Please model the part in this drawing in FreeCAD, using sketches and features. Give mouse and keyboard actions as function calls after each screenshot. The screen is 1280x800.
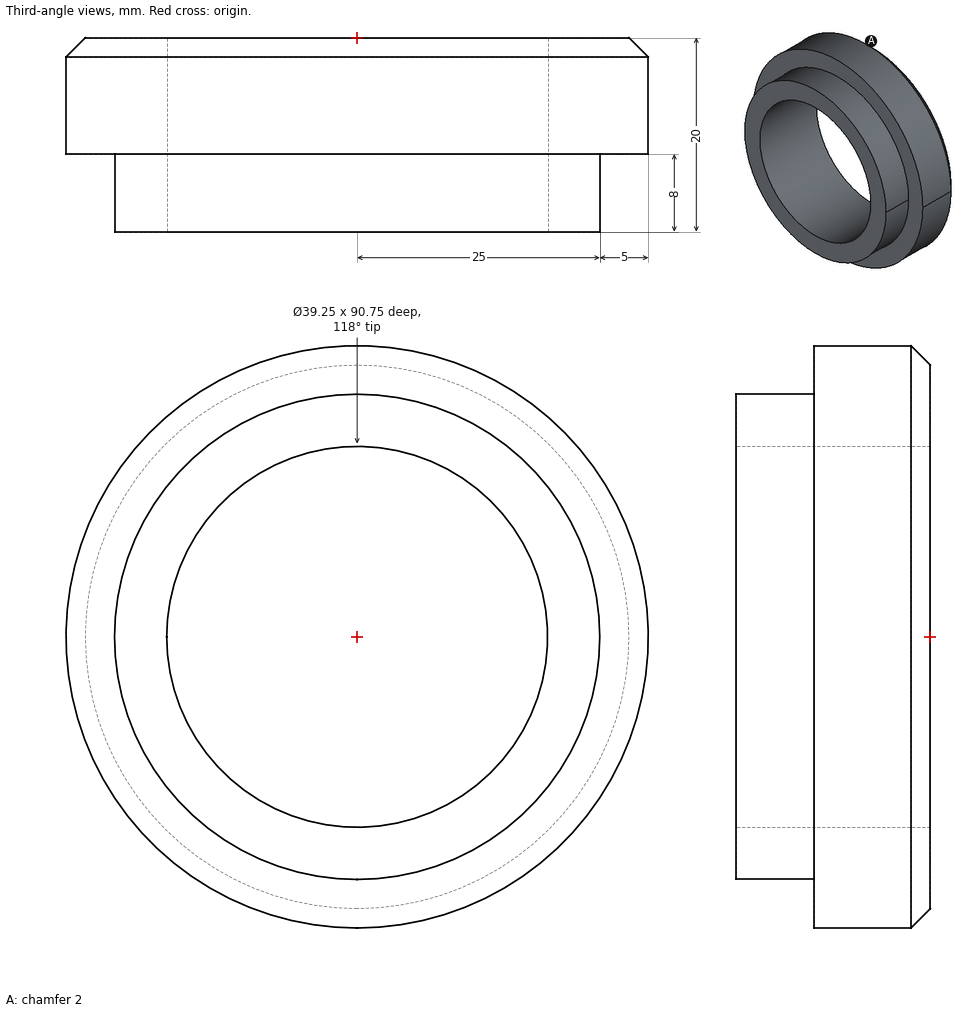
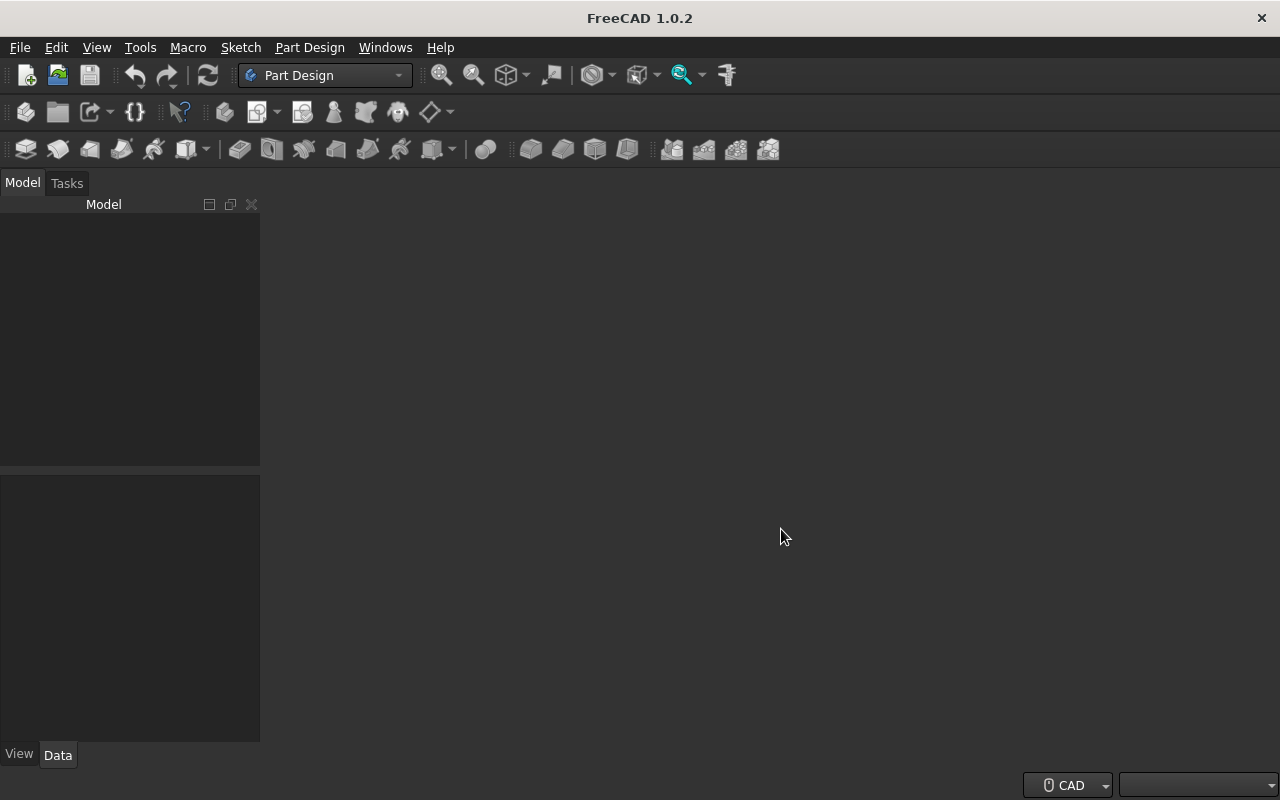
click(26, 76)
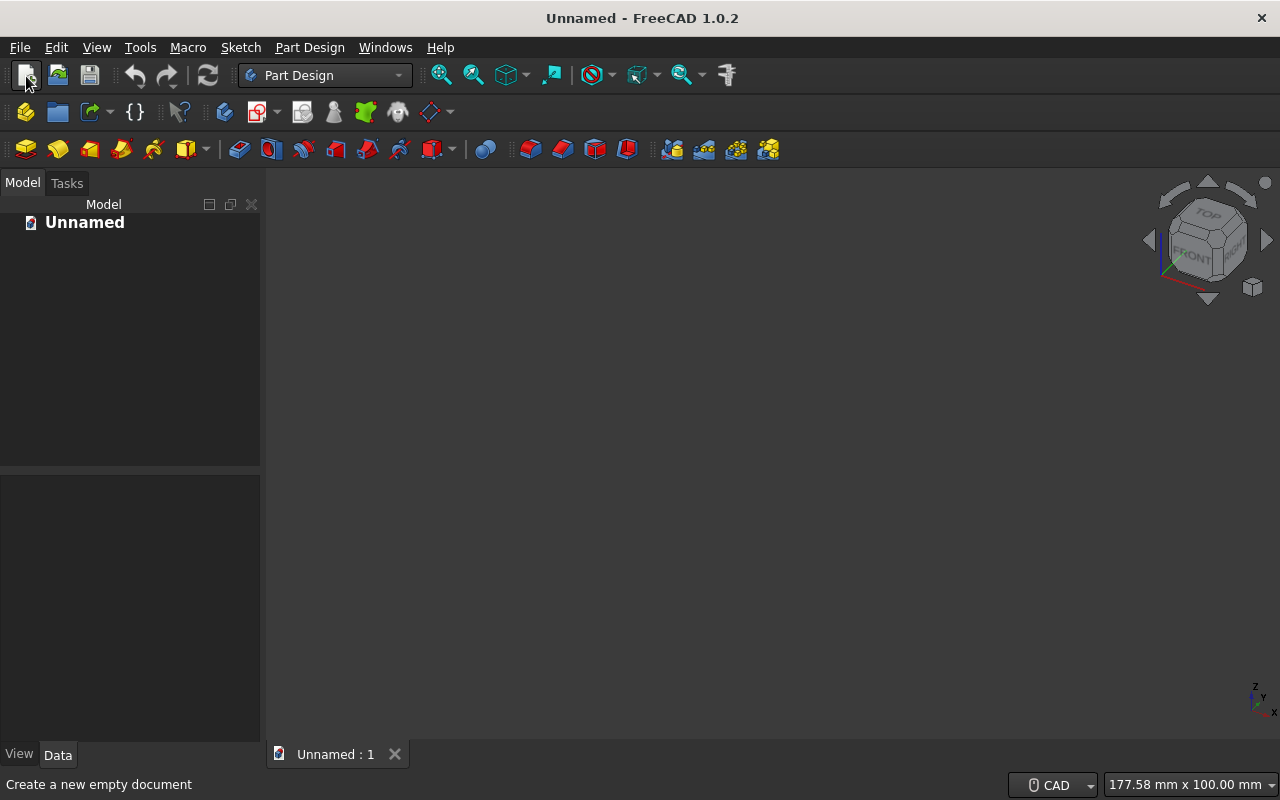
click(258, 112)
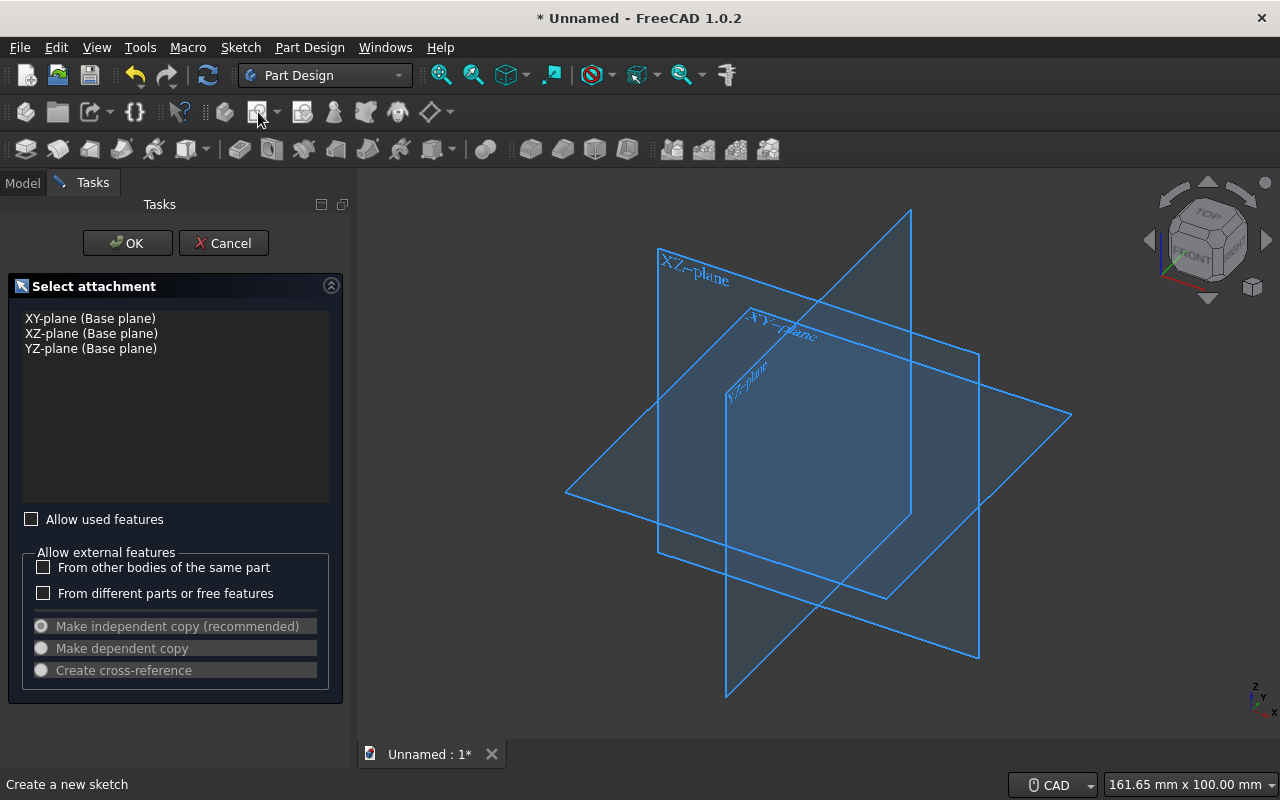
click(82, 318)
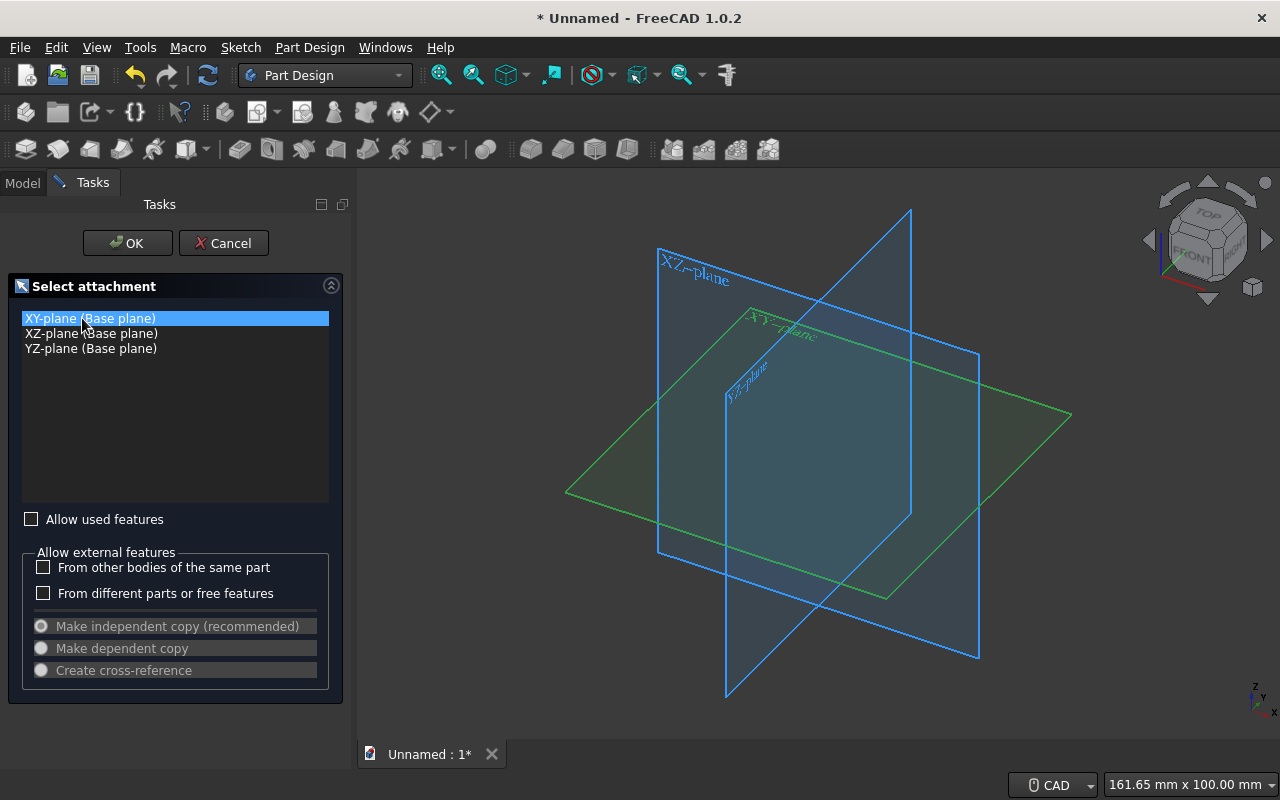
click(128, 243)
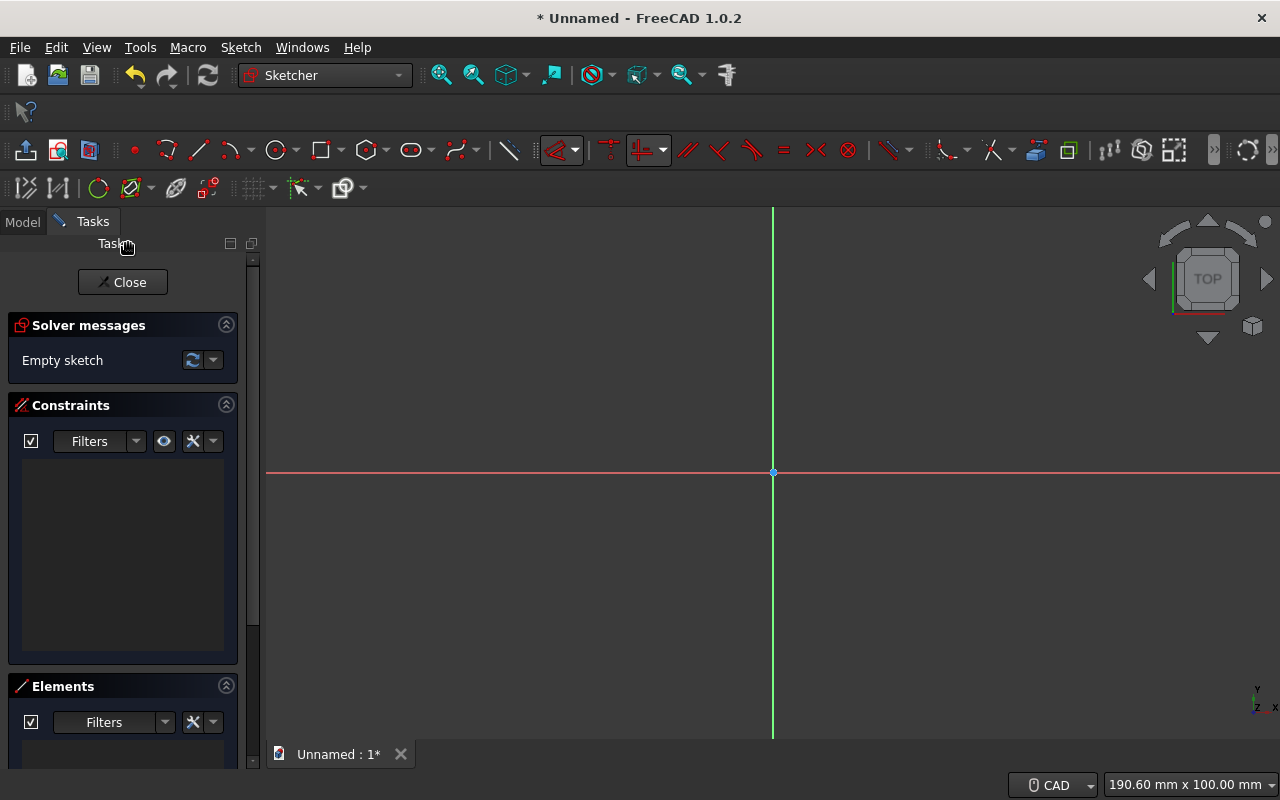
scroll(917, 549, up, 6)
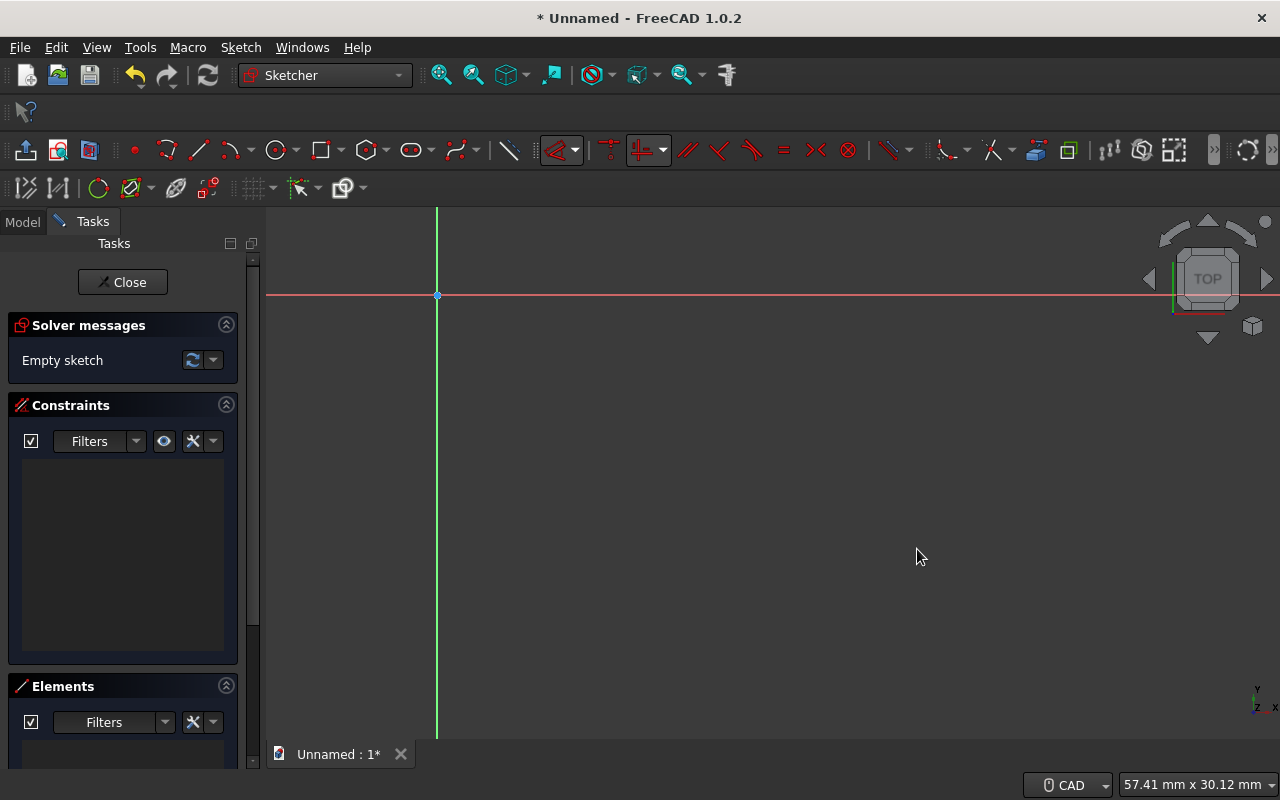
click(168, 150)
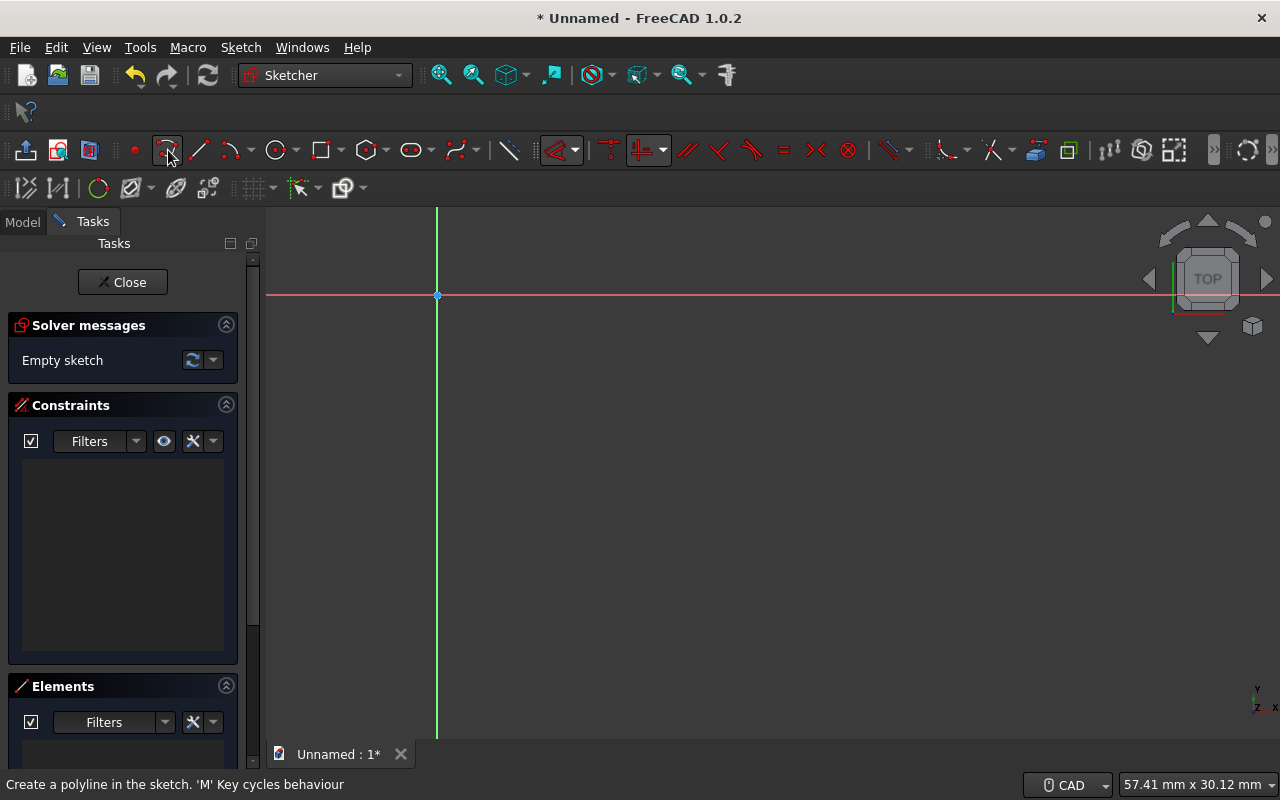
click(437, 295)
click(446, 648)
click(879, 648)
click(879, 507)
click(967, 507)
click(967, 304)
click(437, 295)
key(Escape)
key(Escape)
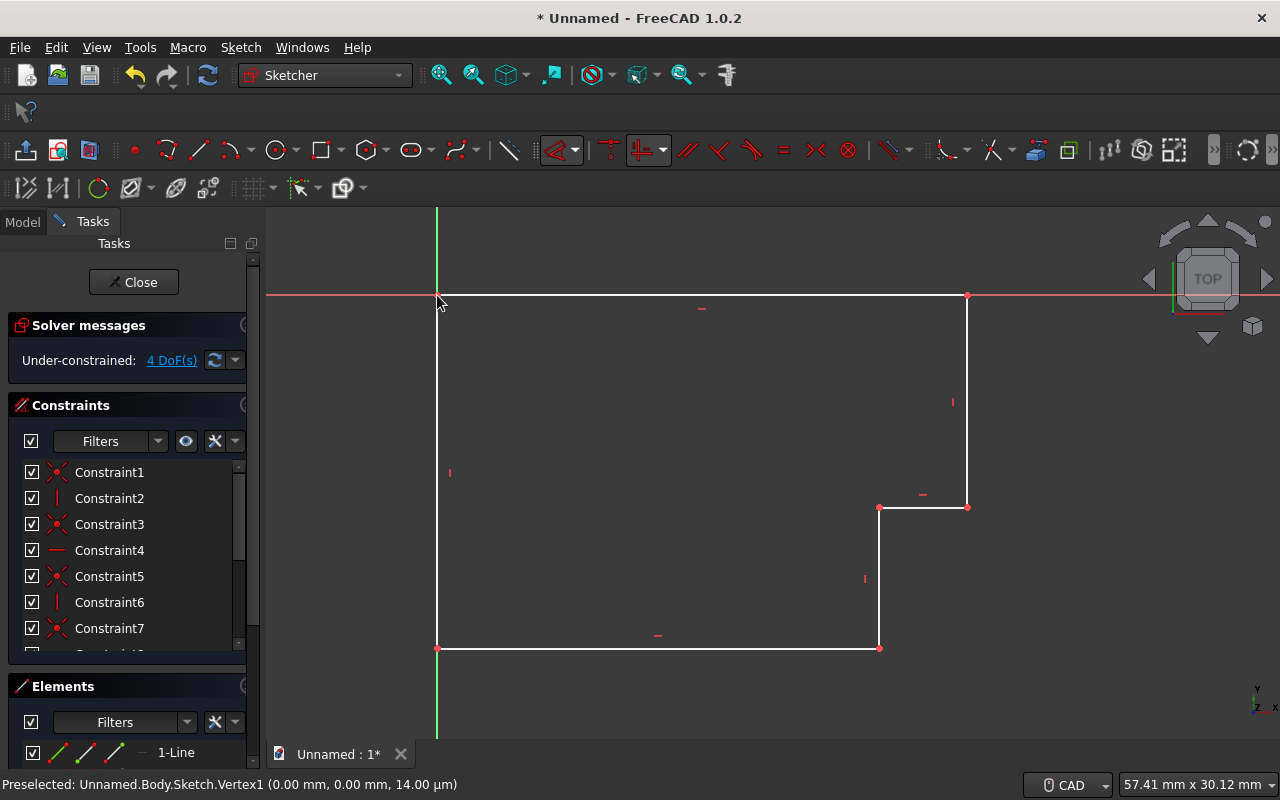
click(879, 607)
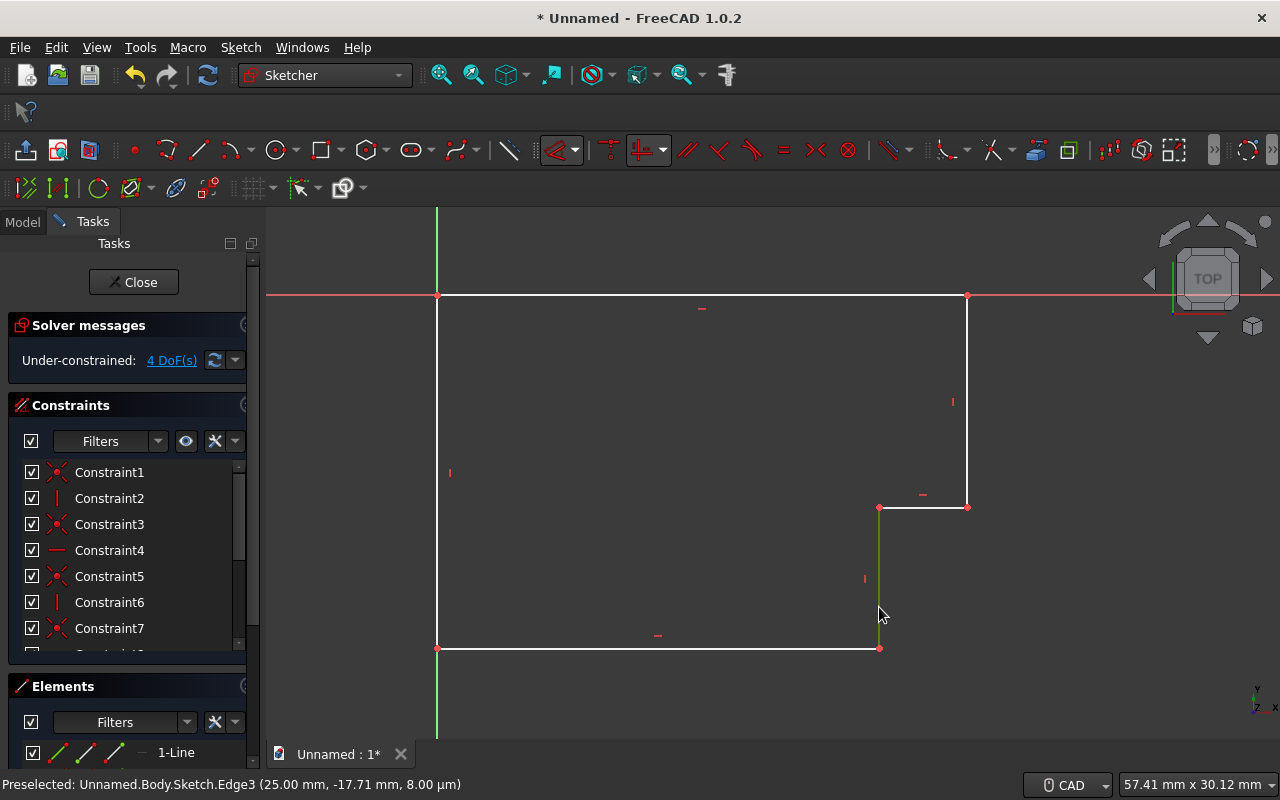
key(i)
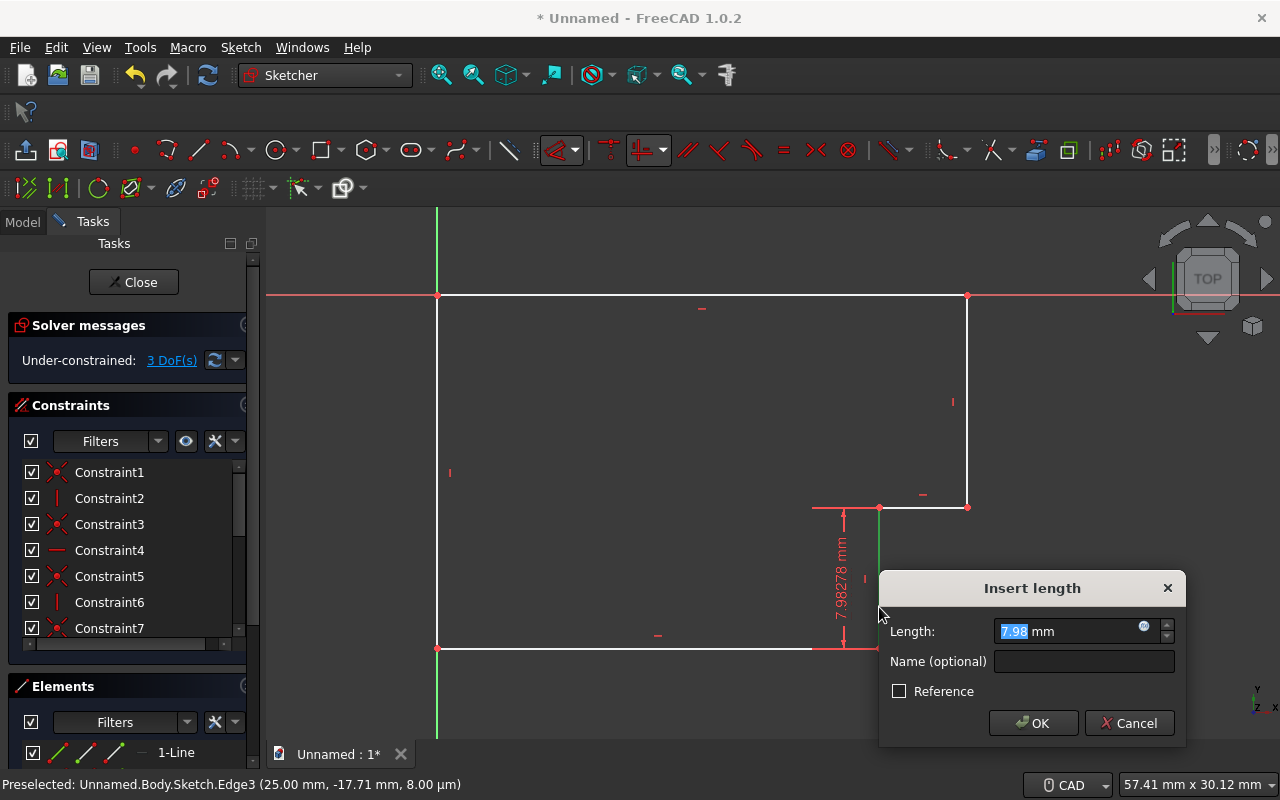
text(8)
key(Return)